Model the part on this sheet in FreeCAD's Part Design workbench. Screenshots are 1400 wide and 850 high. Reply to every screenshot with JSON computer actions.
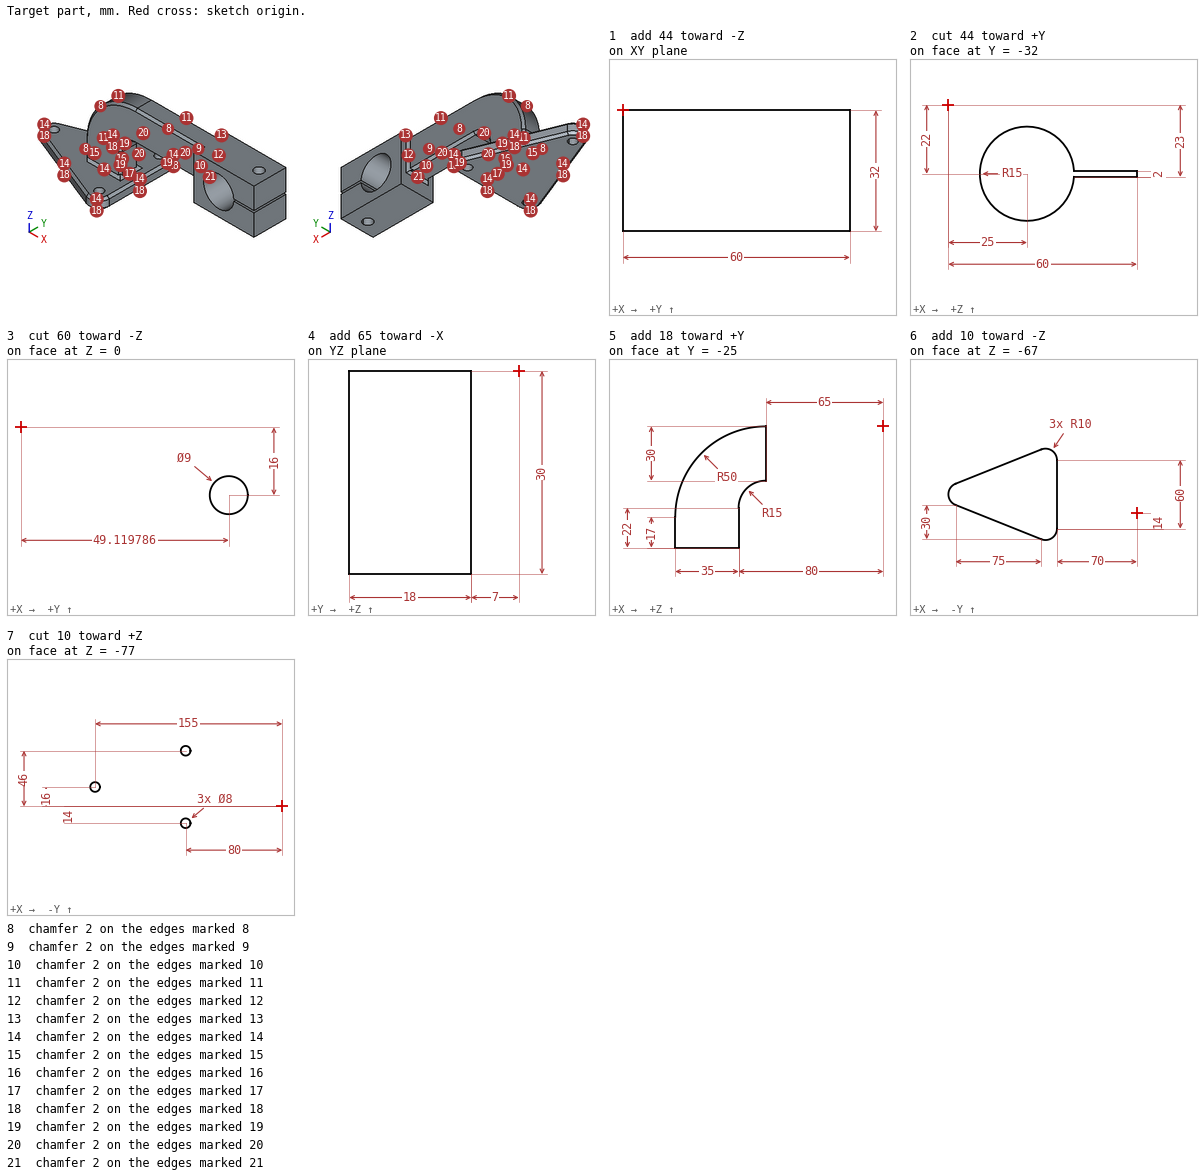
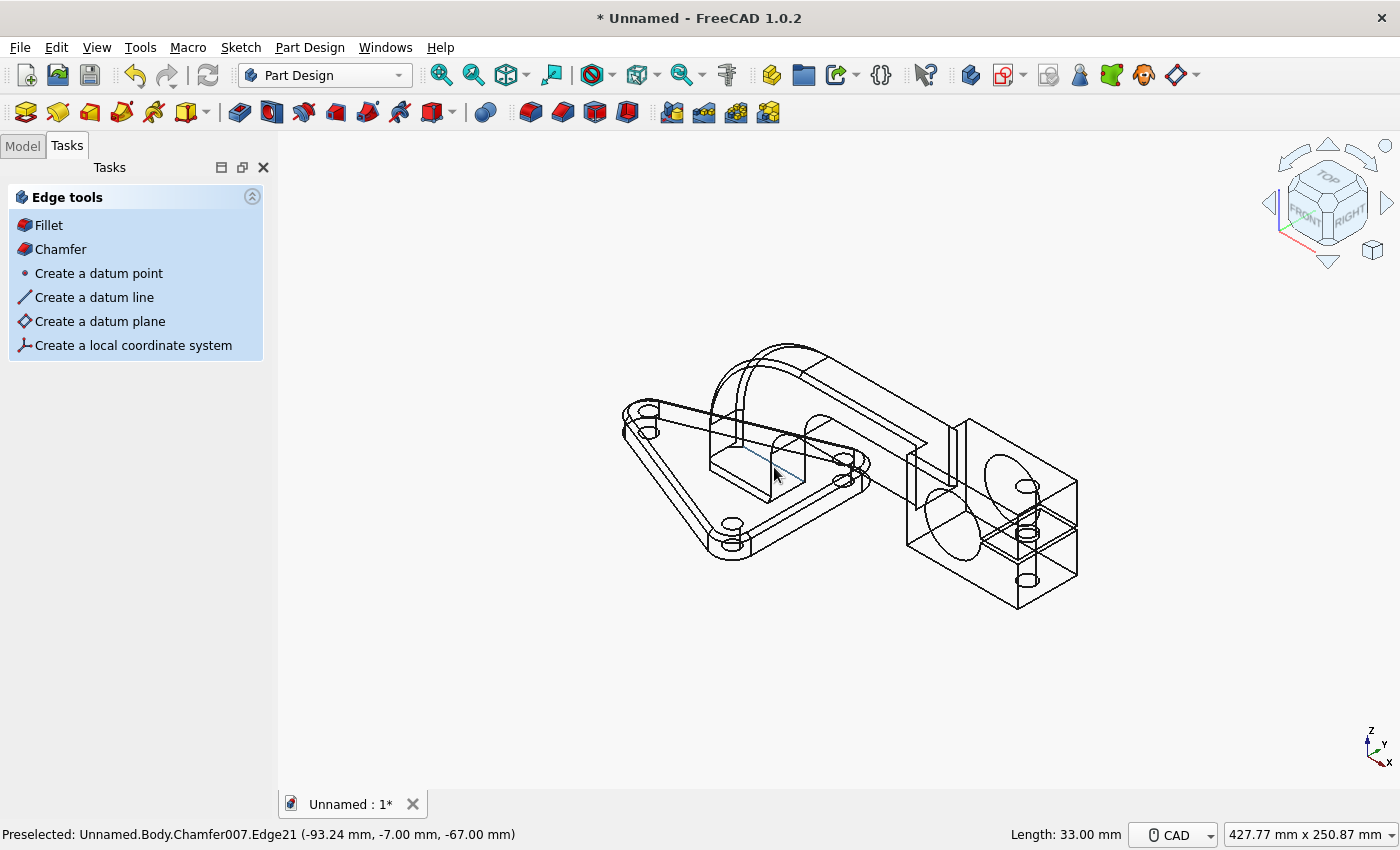
{"action": "left_click", "coordinate": [564, 112]}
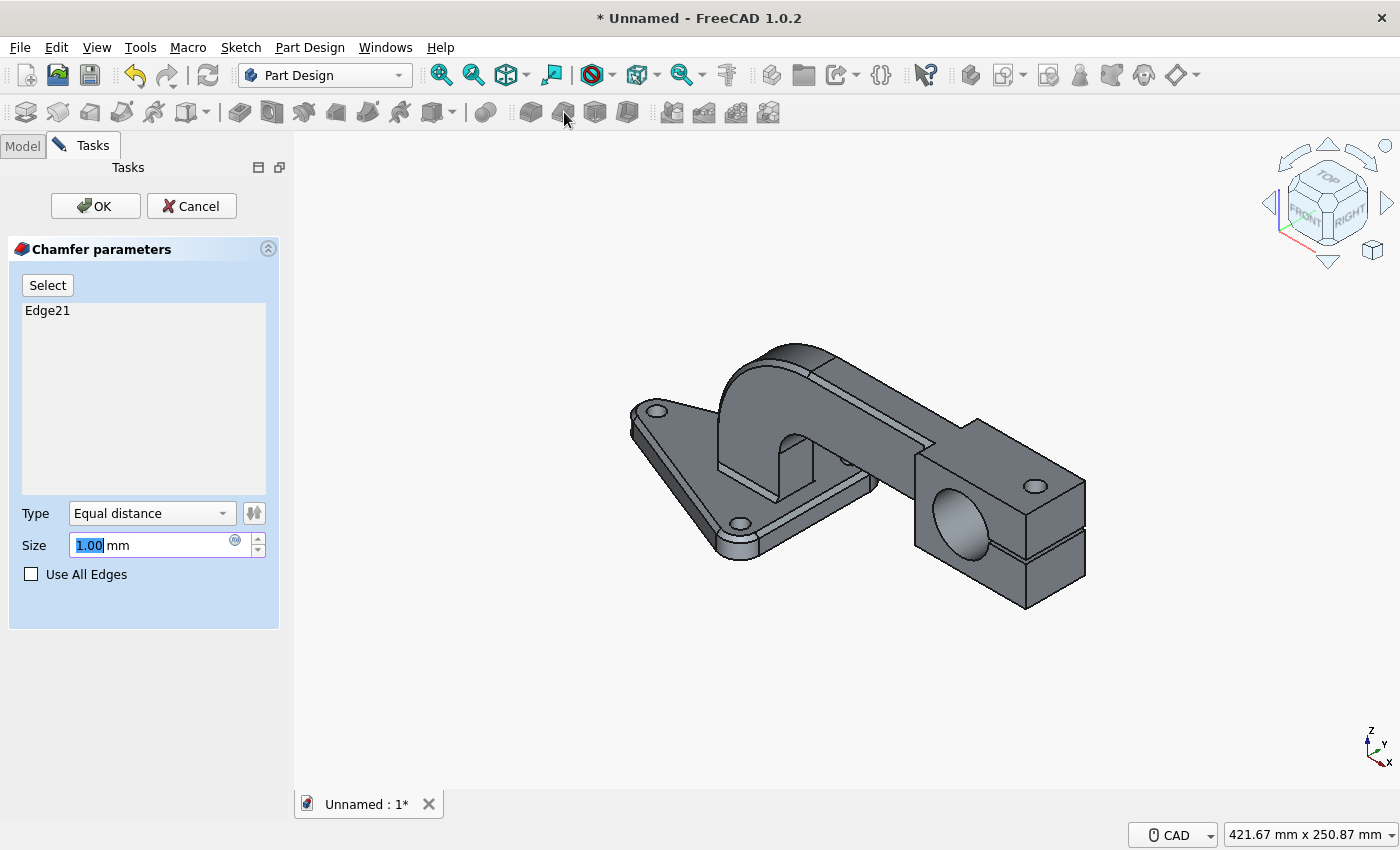
{"action": "type", "text": "2"}
{"action": "key", "text": "Tab"}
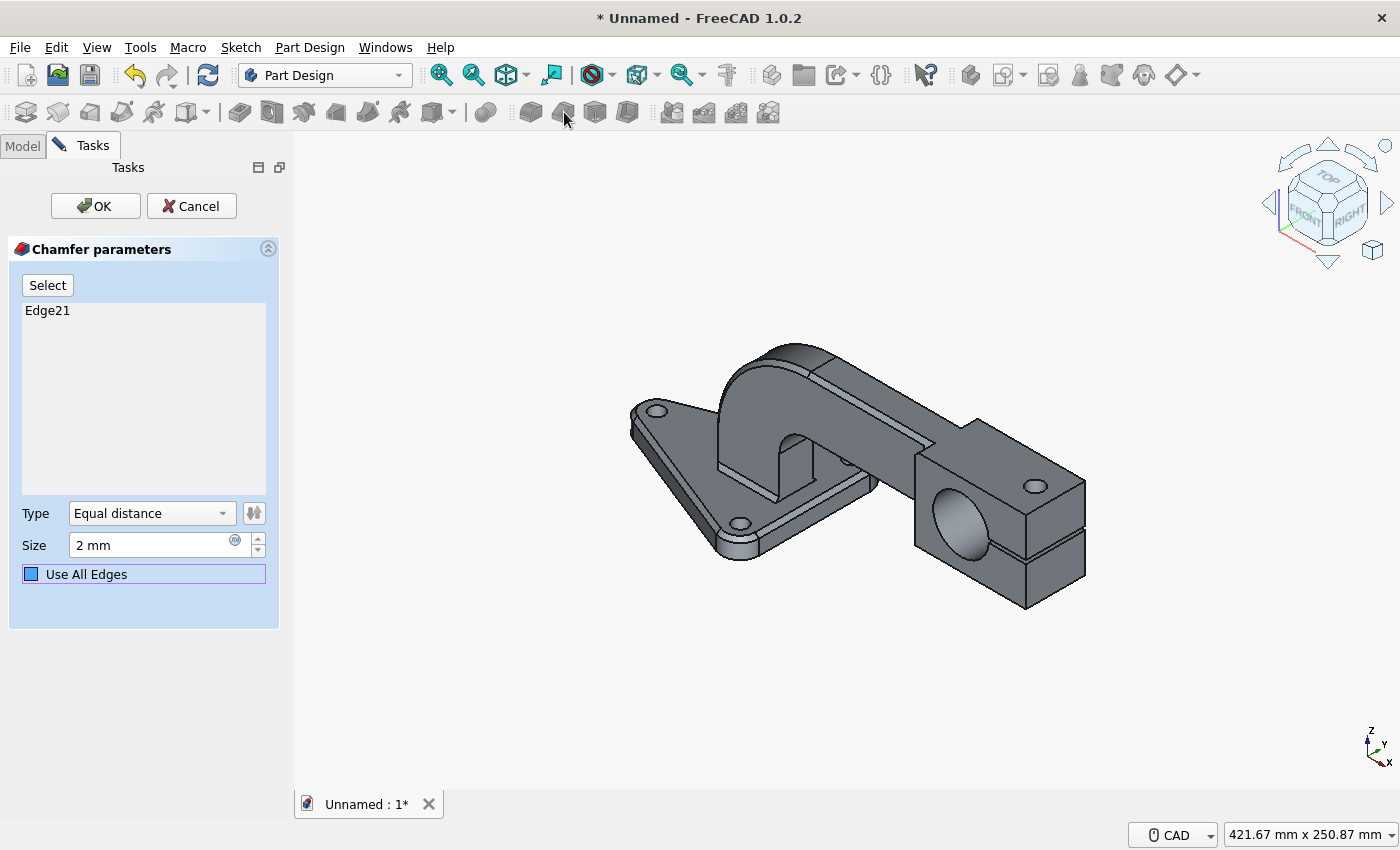
{"action": "left_click", "coordinate": [96, 206]}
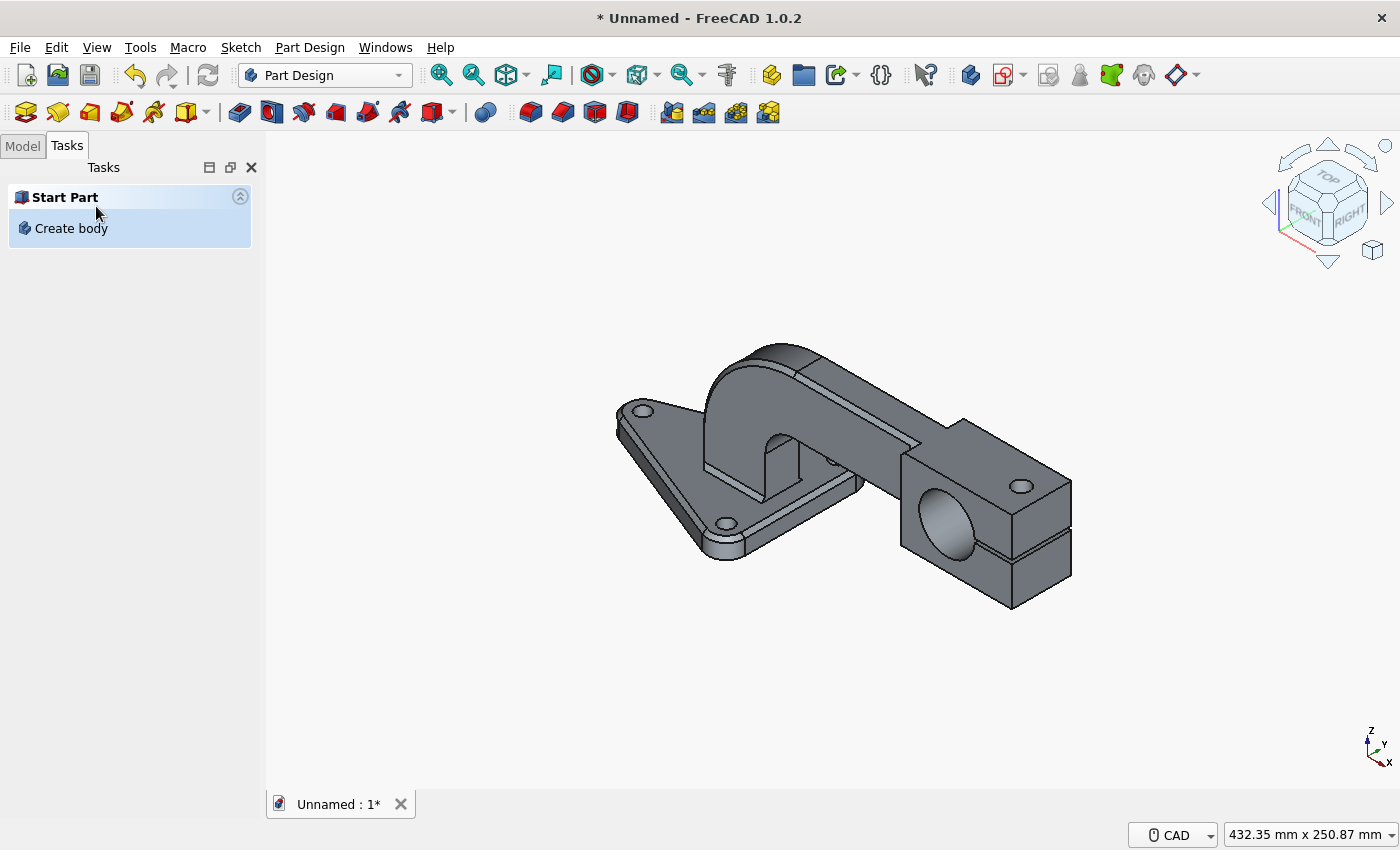
{"action": "key", "text": "2"}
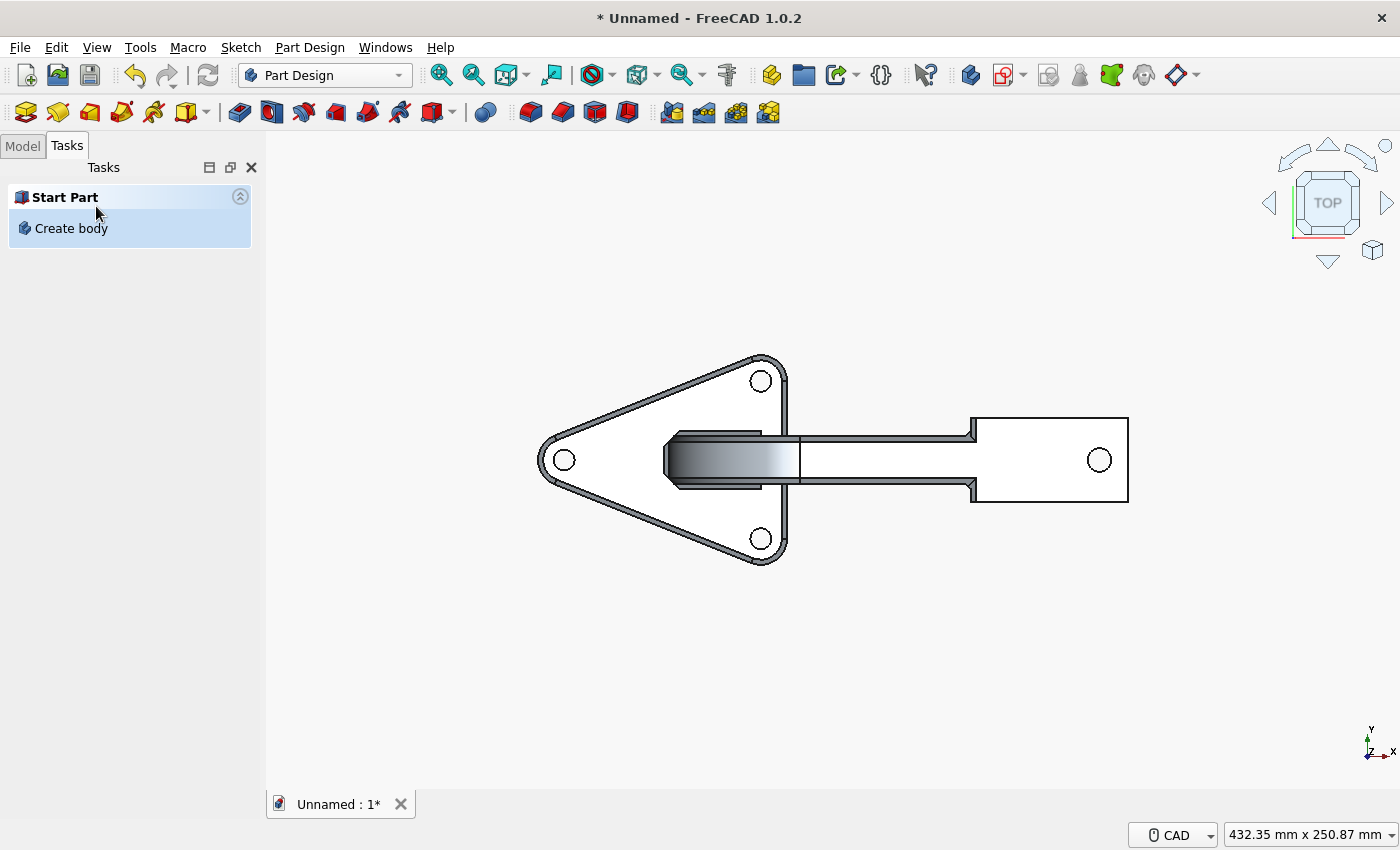
{"action": "key", "text": "0"}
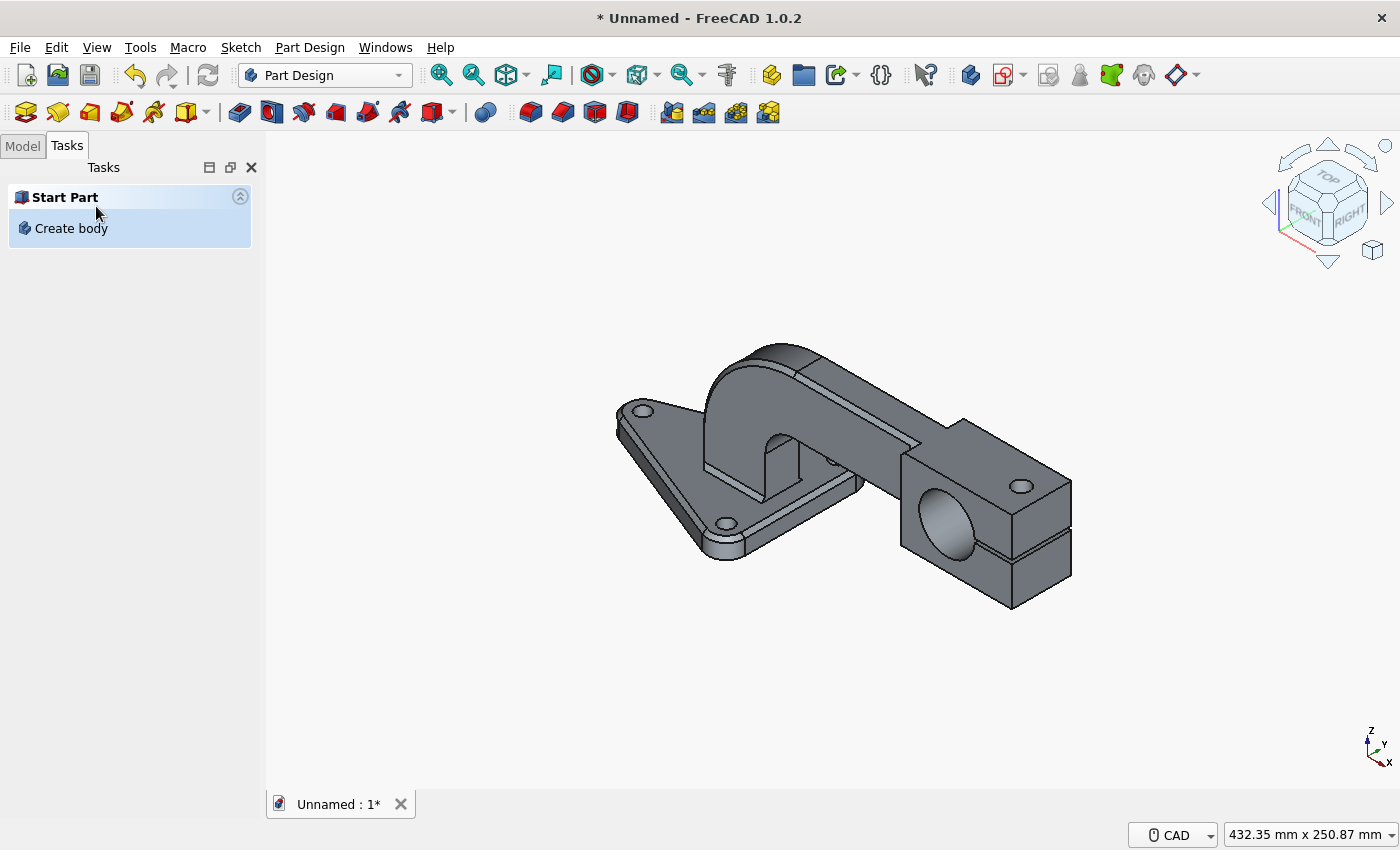
{"action": "key", "text": "1"}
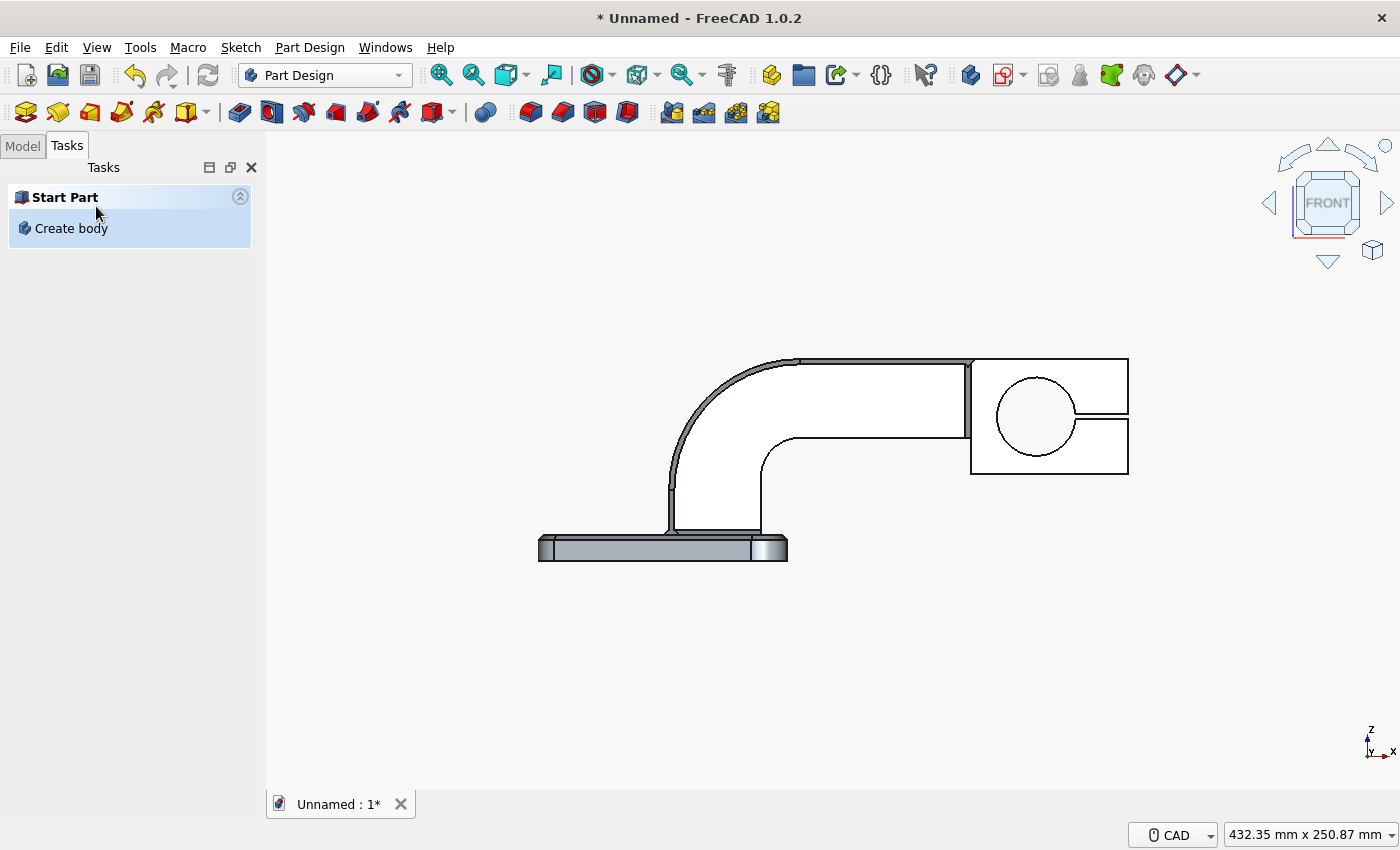
{"action": "key", "text": "3"}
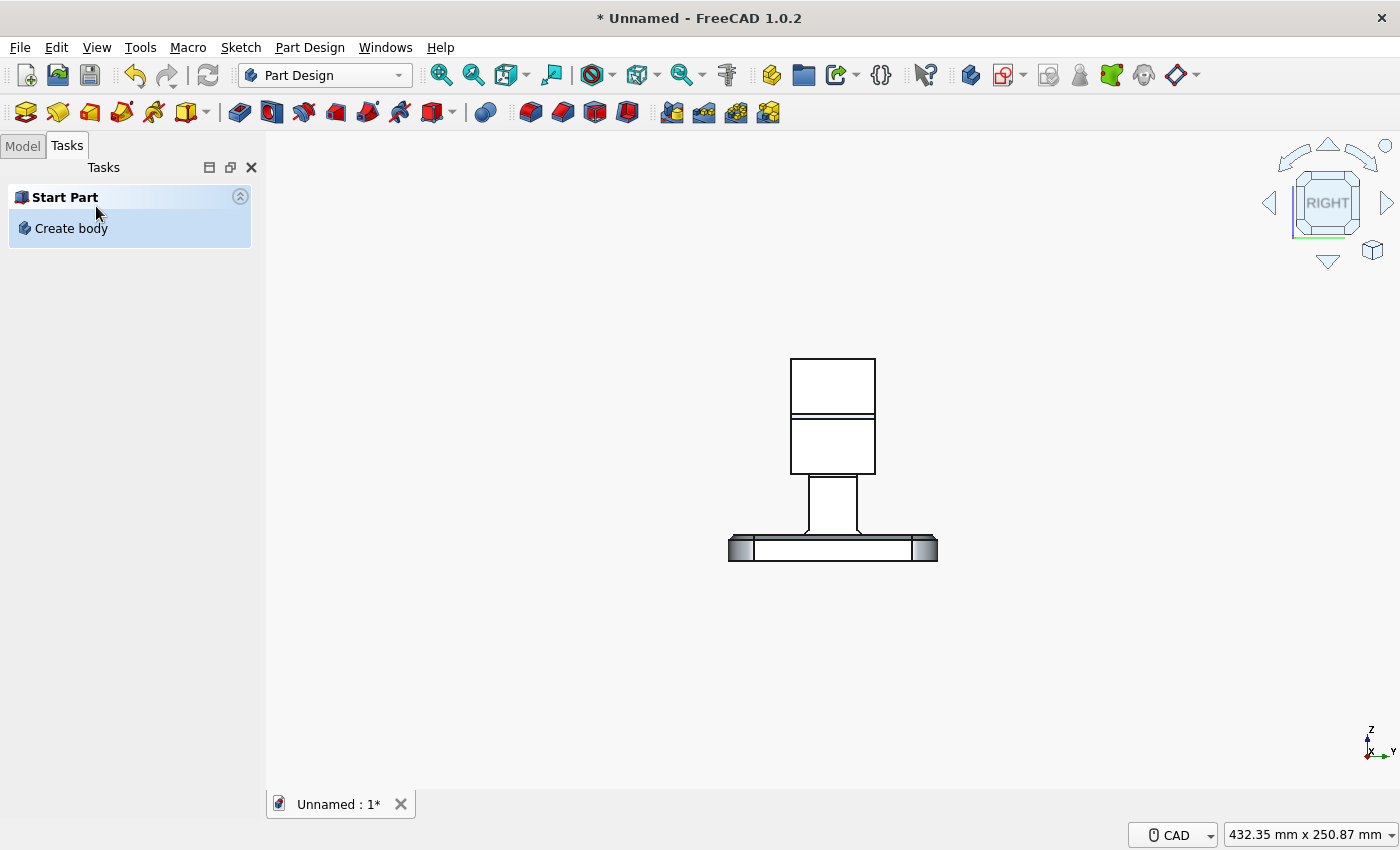
{"action": "left_click", "coordinate": [442, 76]}